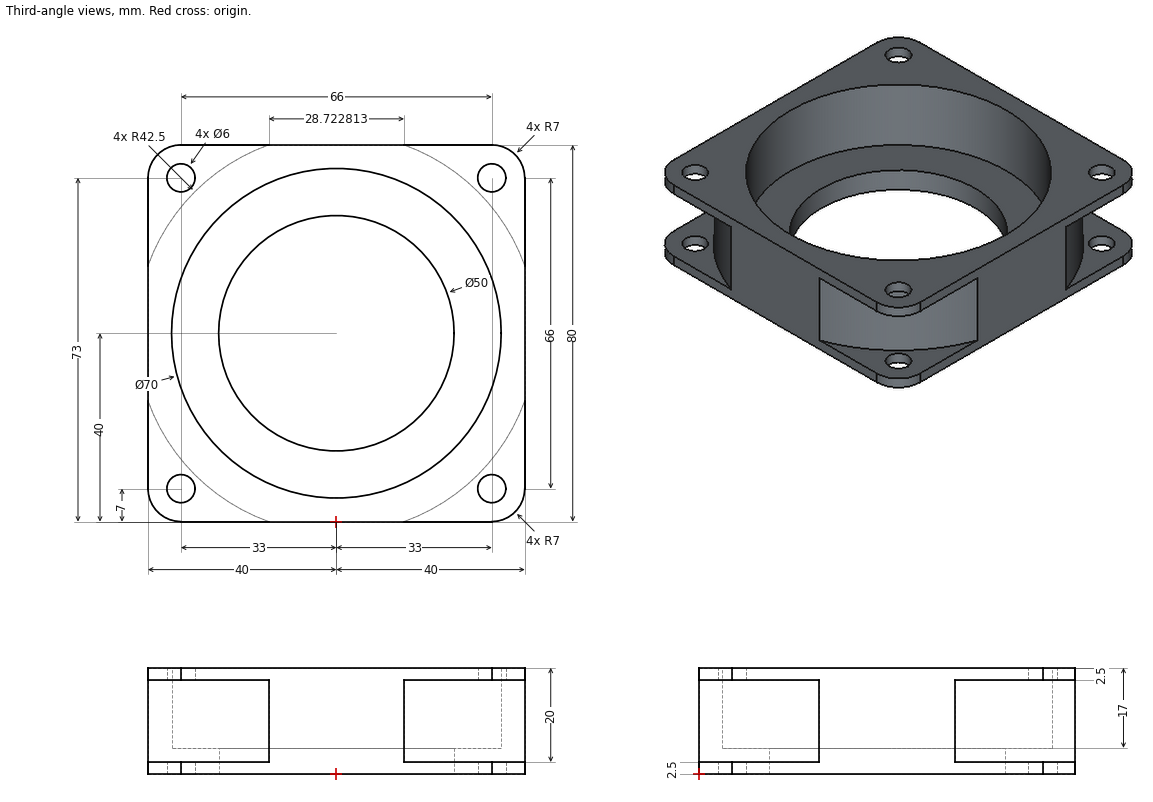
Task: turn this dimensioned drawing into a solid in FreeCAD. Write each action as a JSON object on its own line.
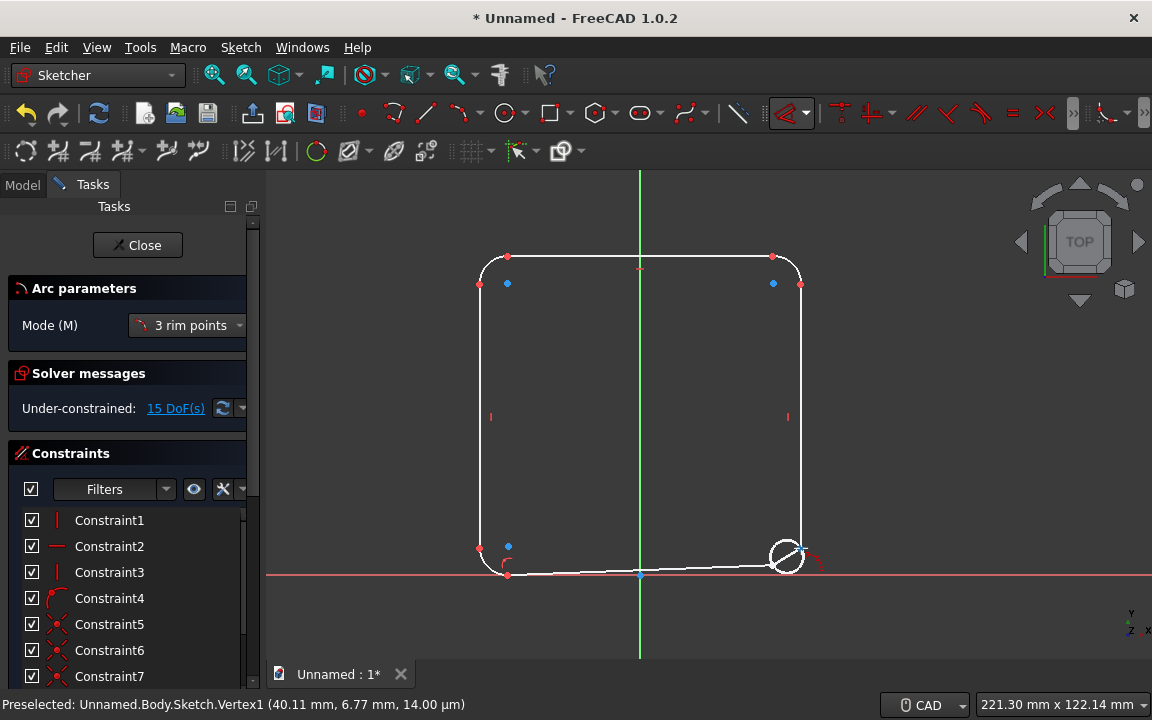
{"action": "scroll", "coordinate": [792, 567], "scroll_direction": "up", "scroll_amount": 4}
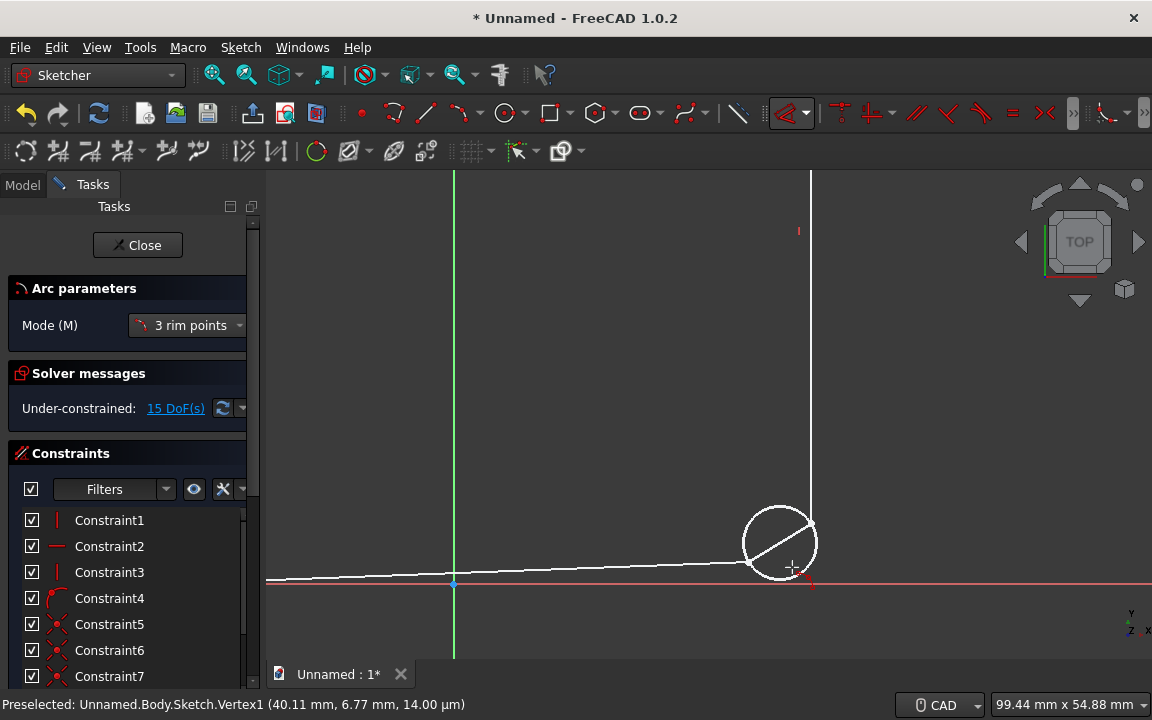
{"action": "left_click", "coordinate": [792, 566]}
{"action": "key", "text": "Escape"}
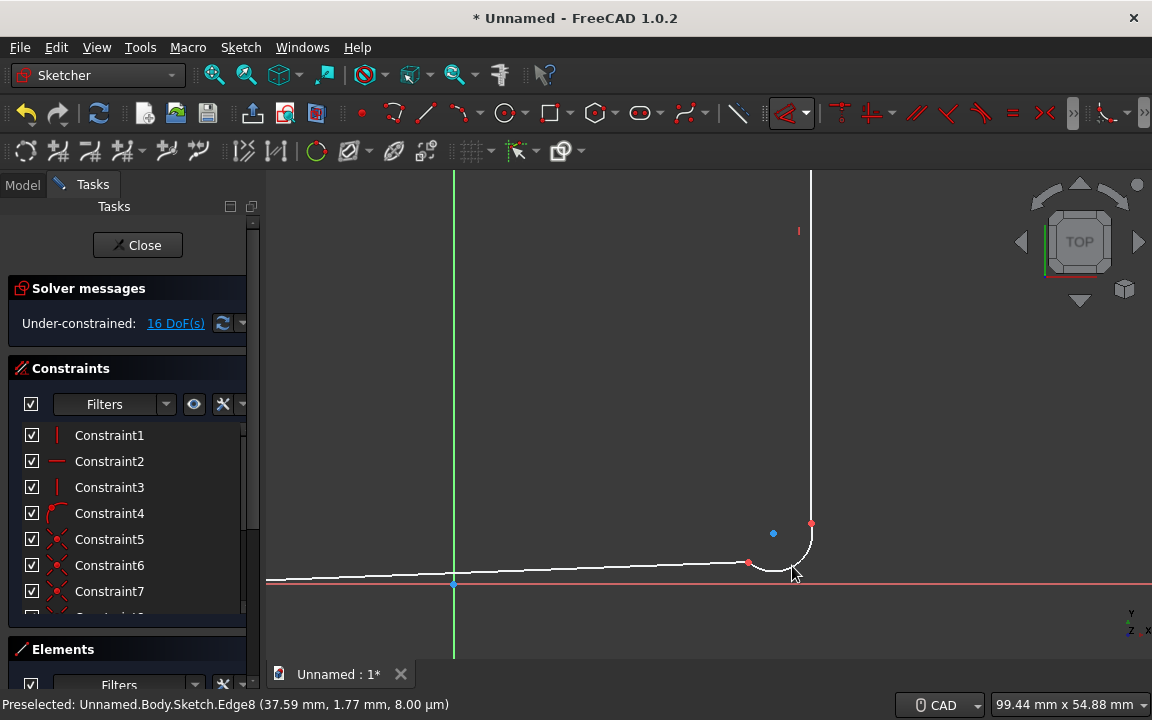
{"action": "left_click", "coordinate": [811, 348]}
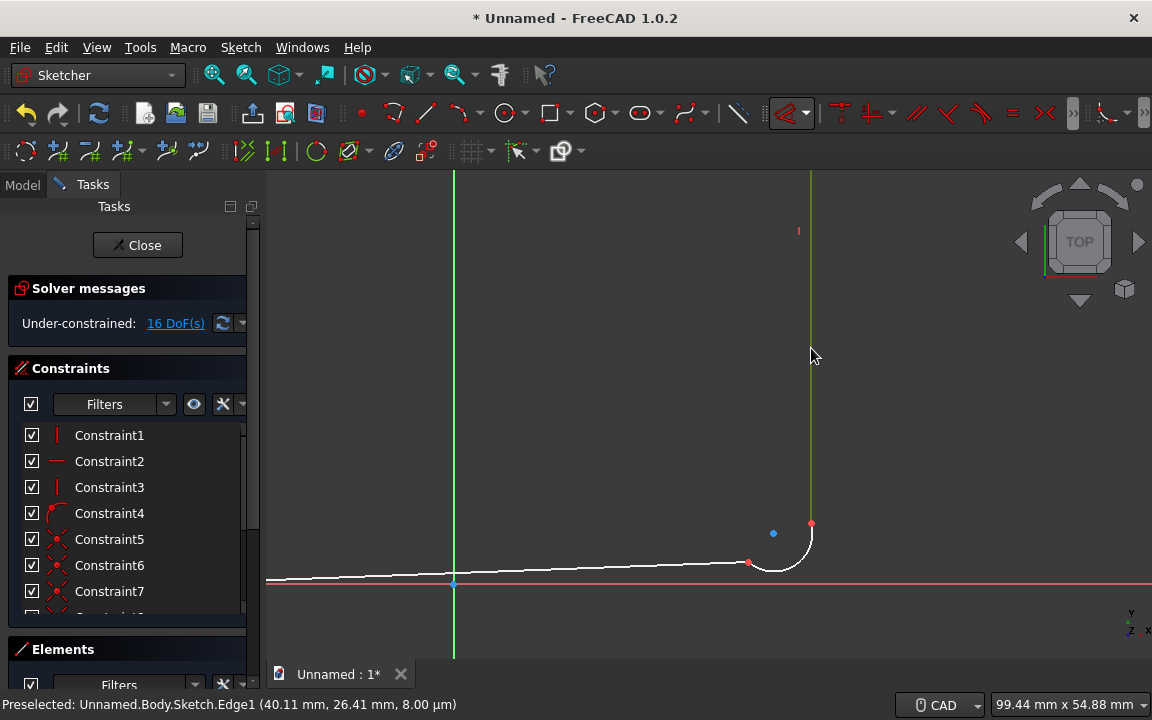
{"action": "scroll", "coordinate": [793, 567], "scroll_direction": "down", "scroll_amount": 4}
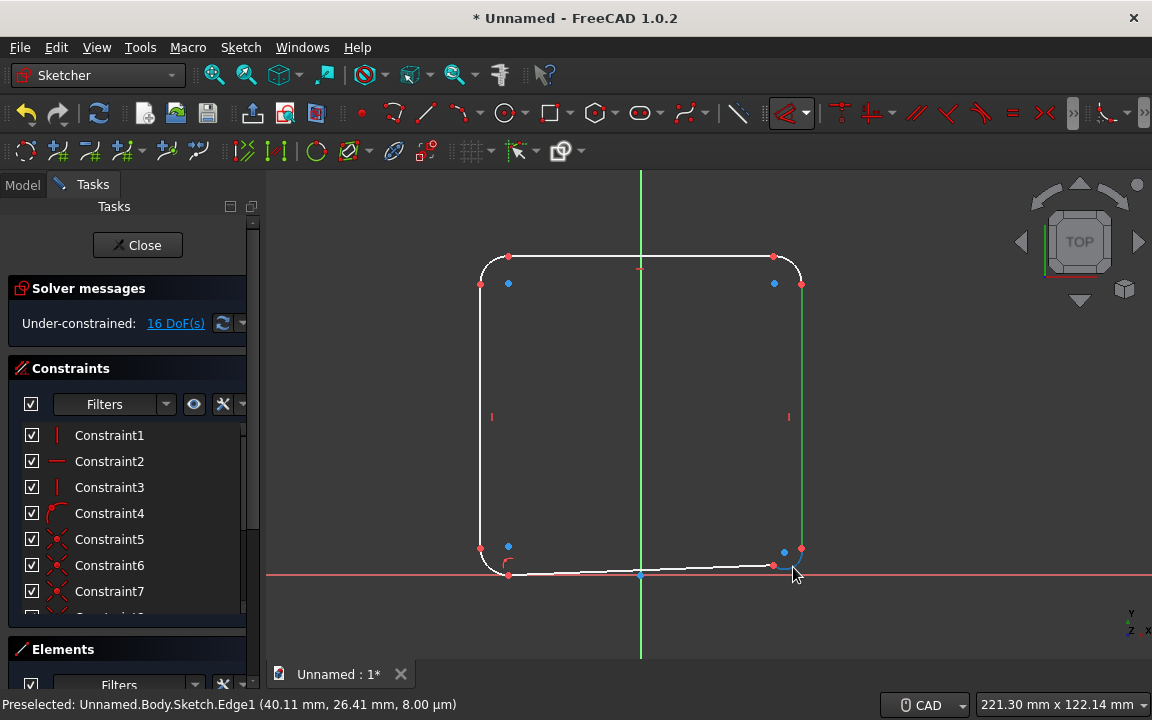
{"action": "left_click", "coordinate": [799, 271]}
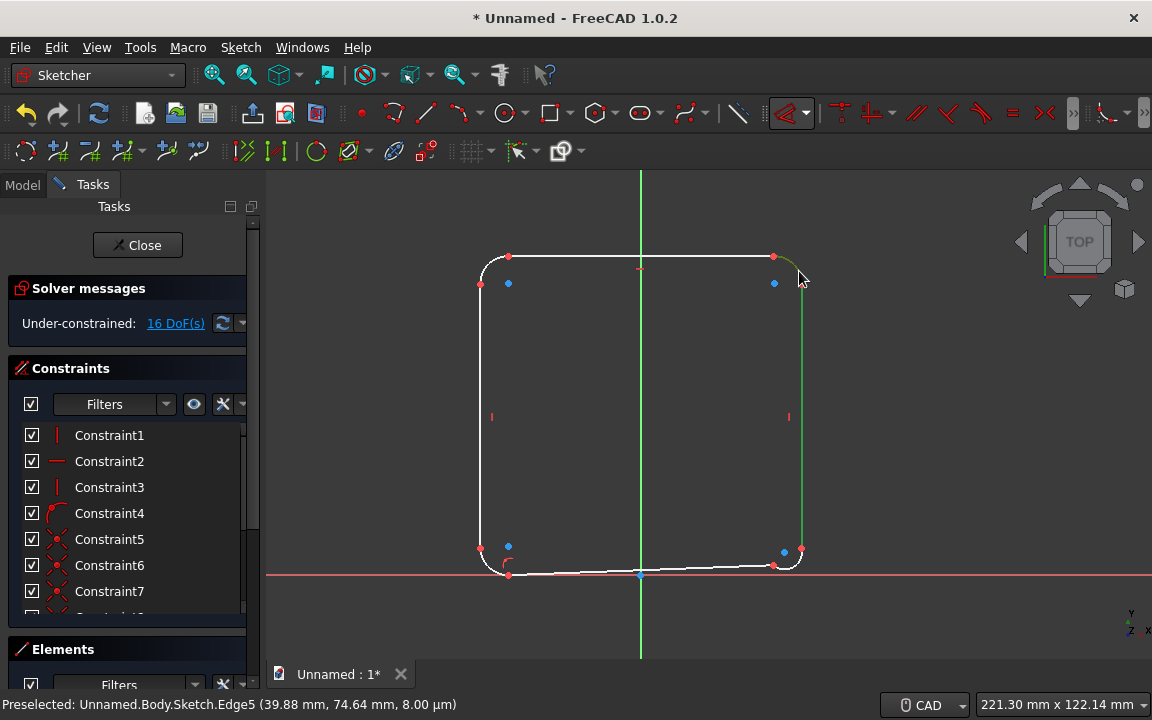
{"action": "left_click", "coordinate": [982, 114]}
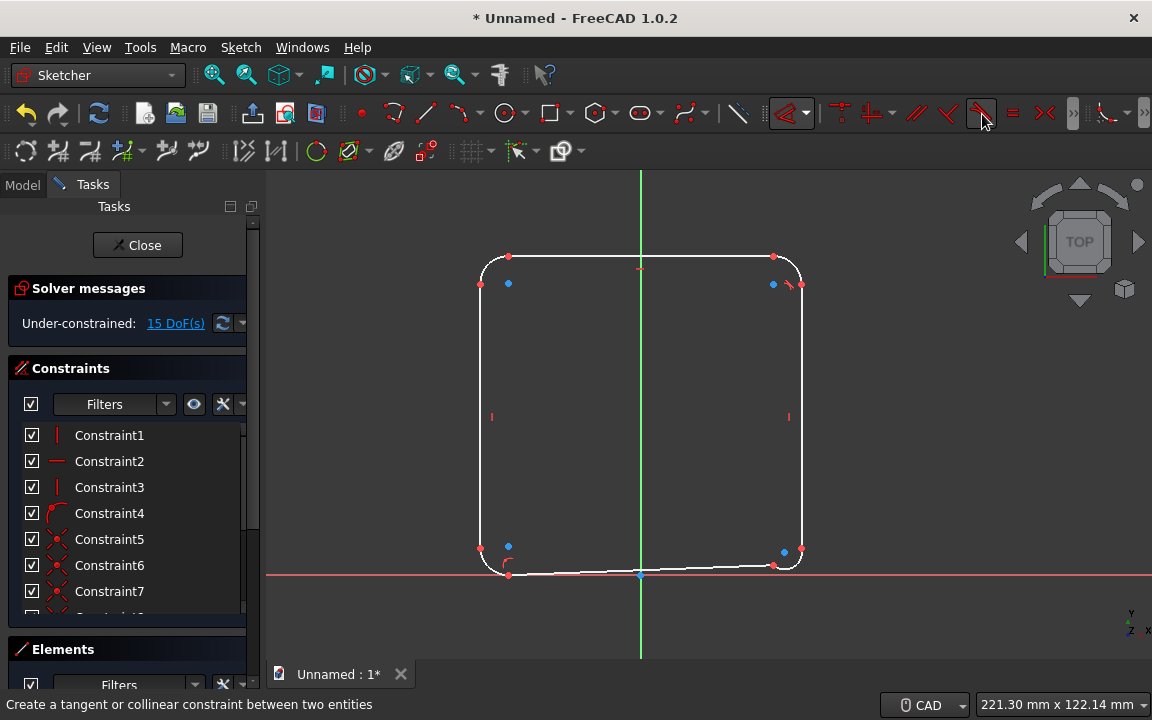
{"action": "left_click", "coordinate": [802, 469]}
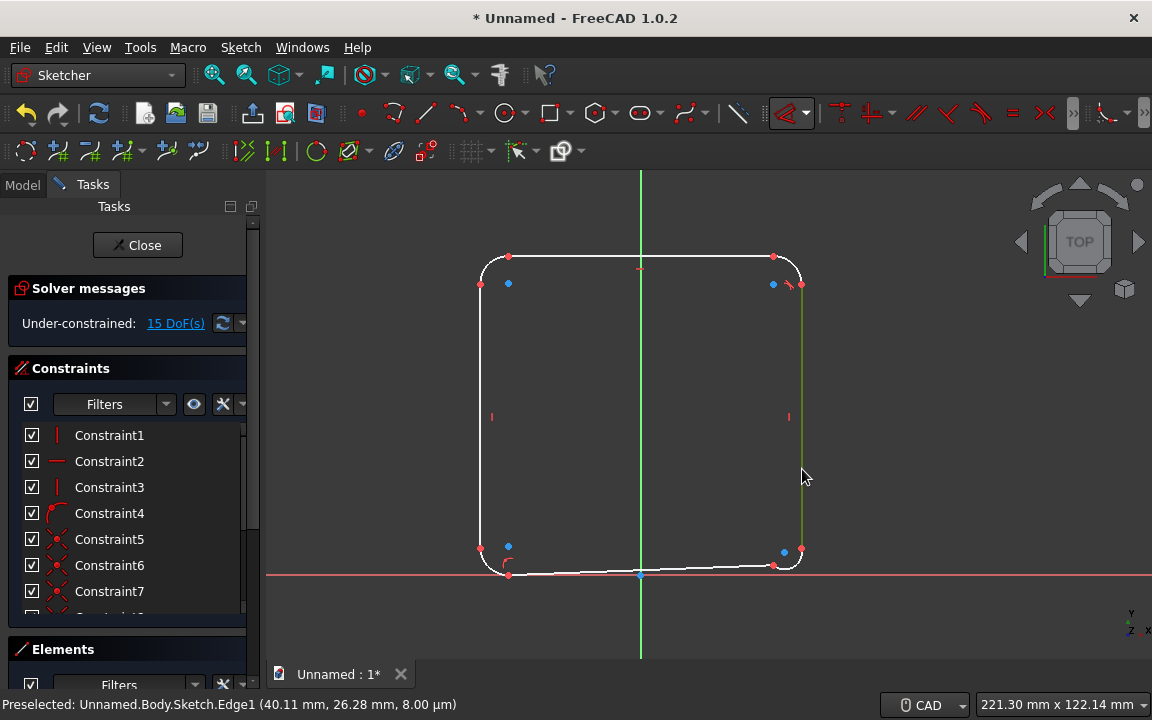
{"action": "left_click", "coordinate": [800, 561]}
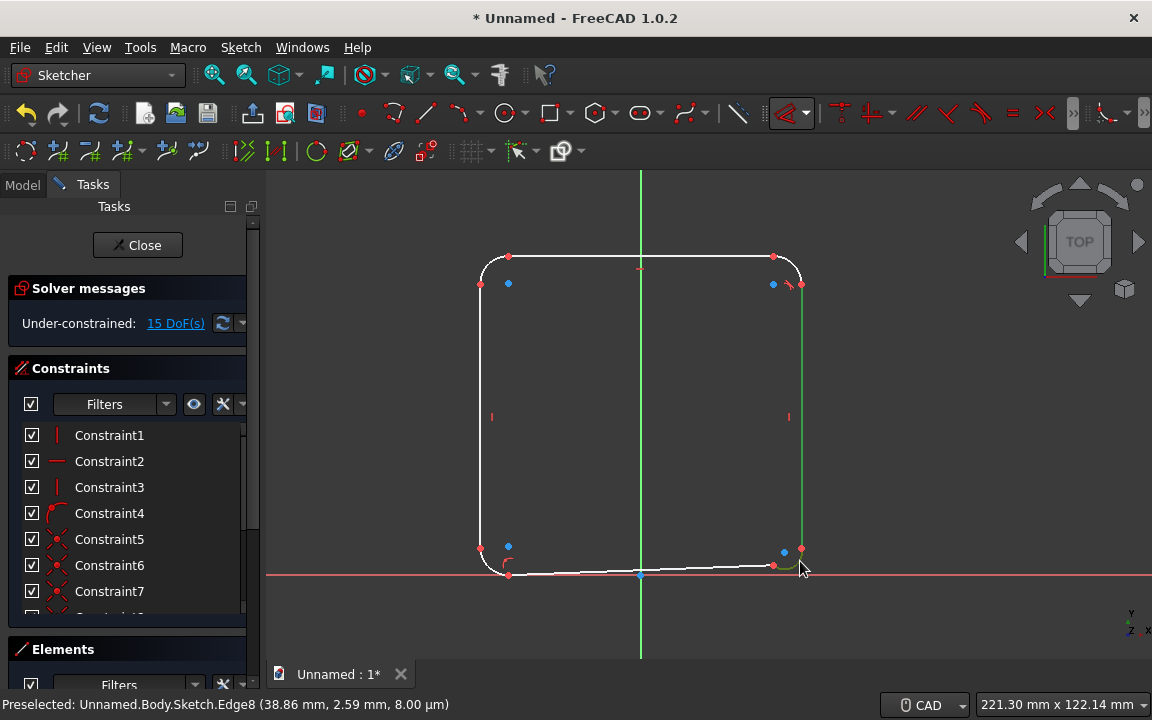
{"action": "key", "text": "t"}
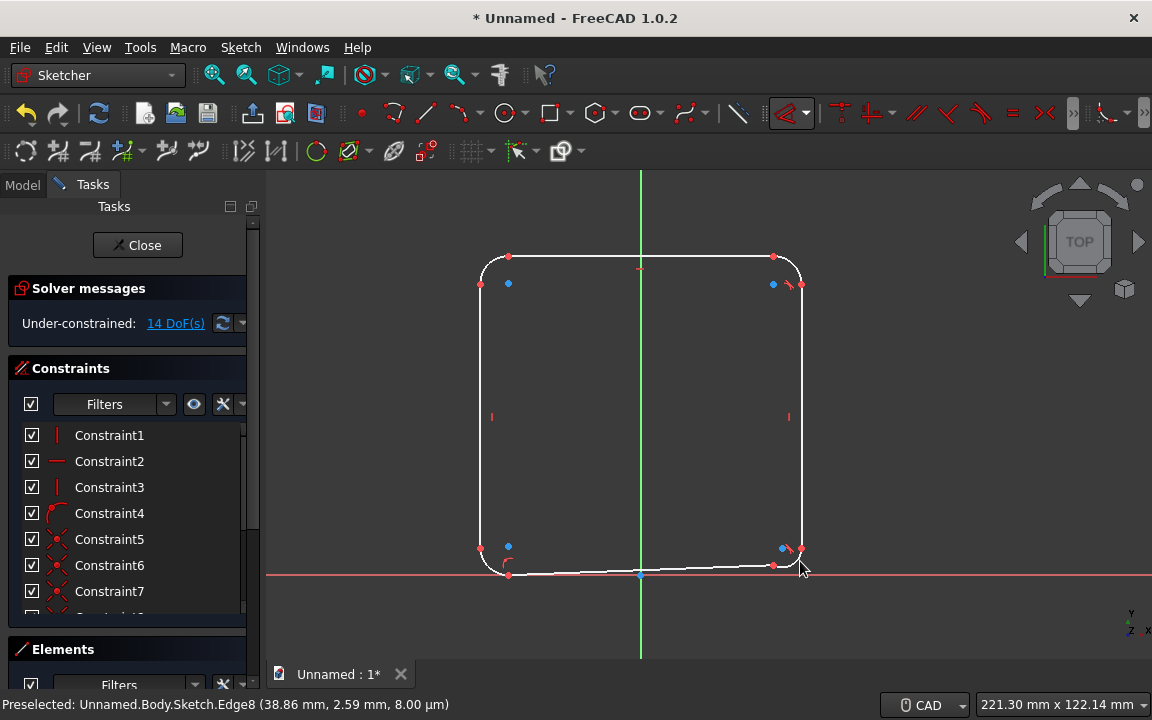
{"action": "left_click", "coordinate": [694, 256]}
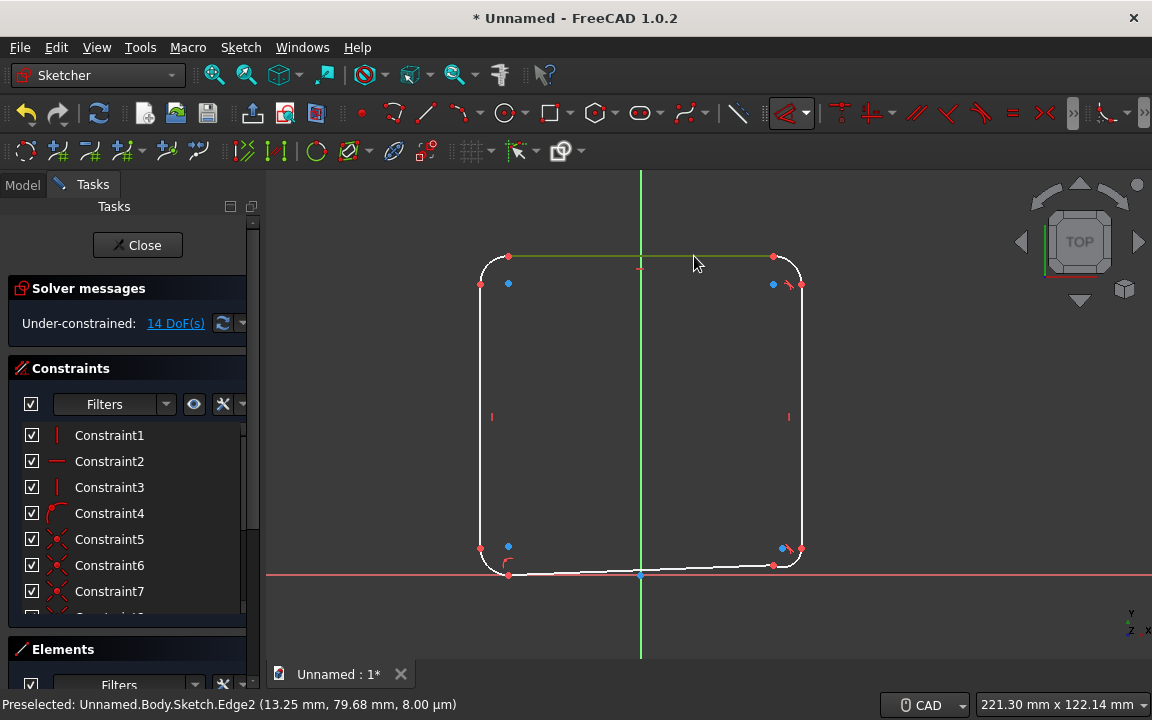
{"action": "left_click", "coordinate": [798, 272]}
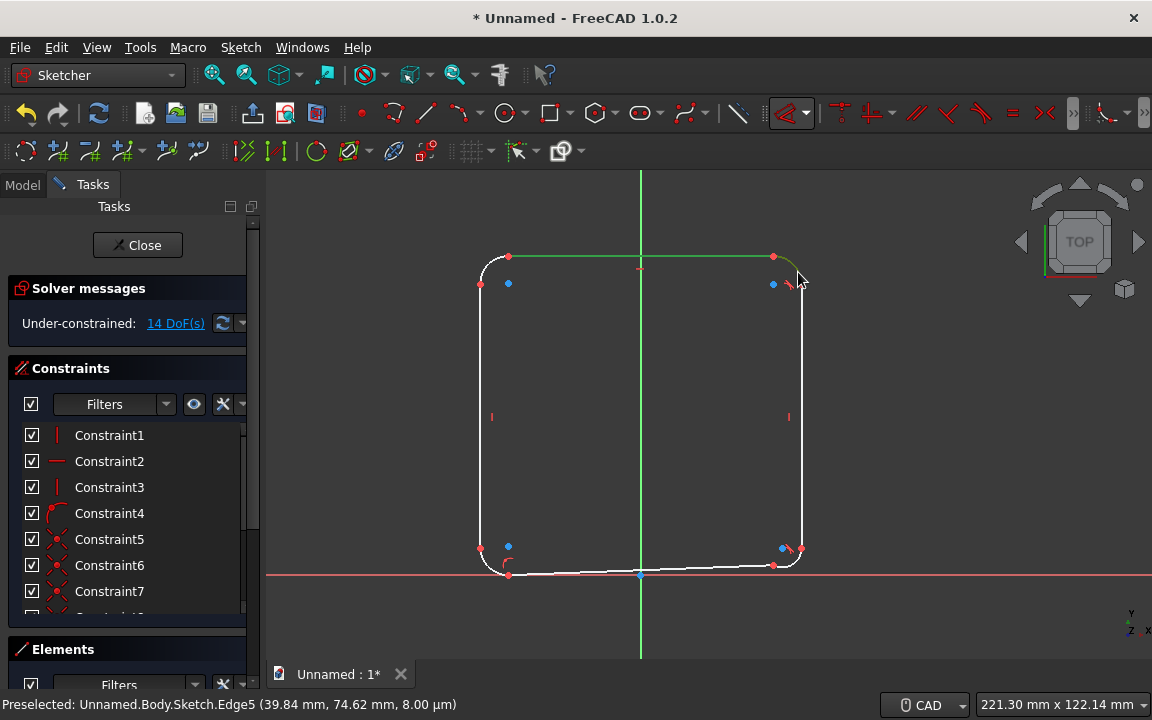
{"action": "left_click", "coordinate": [982, 114]}